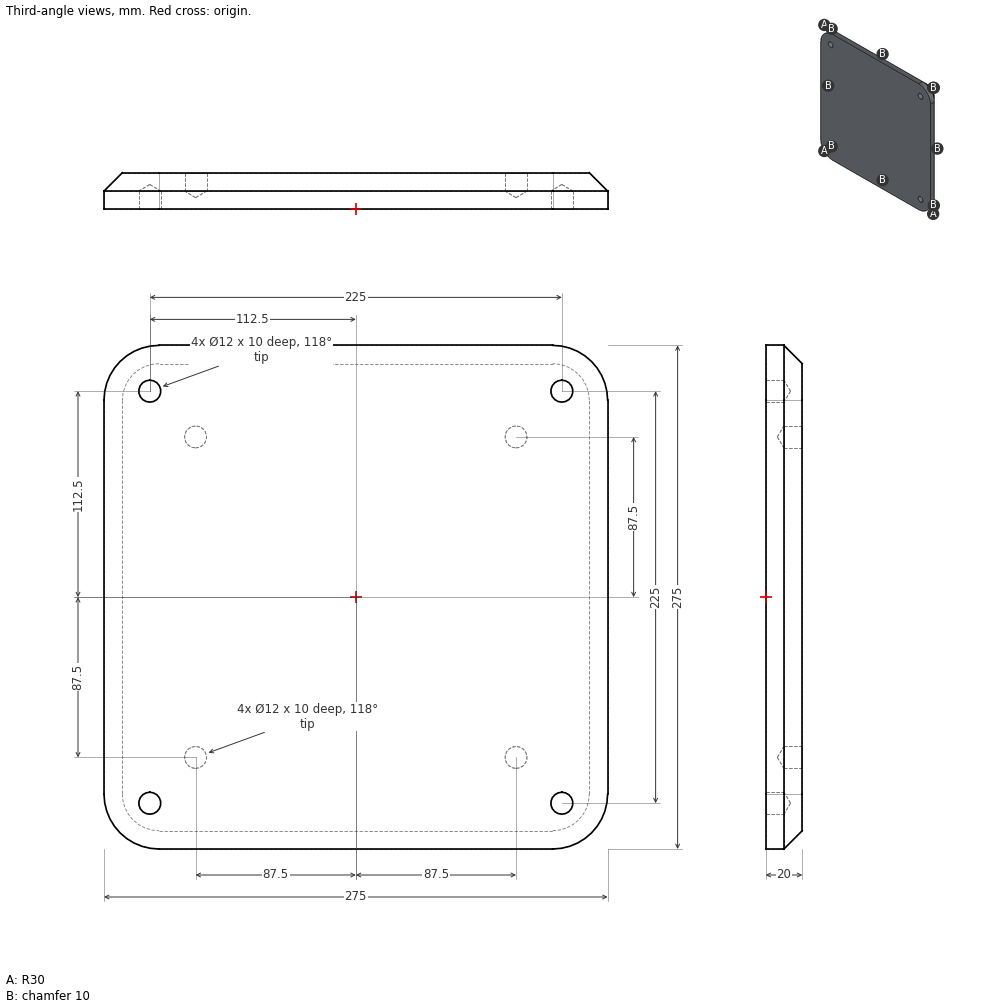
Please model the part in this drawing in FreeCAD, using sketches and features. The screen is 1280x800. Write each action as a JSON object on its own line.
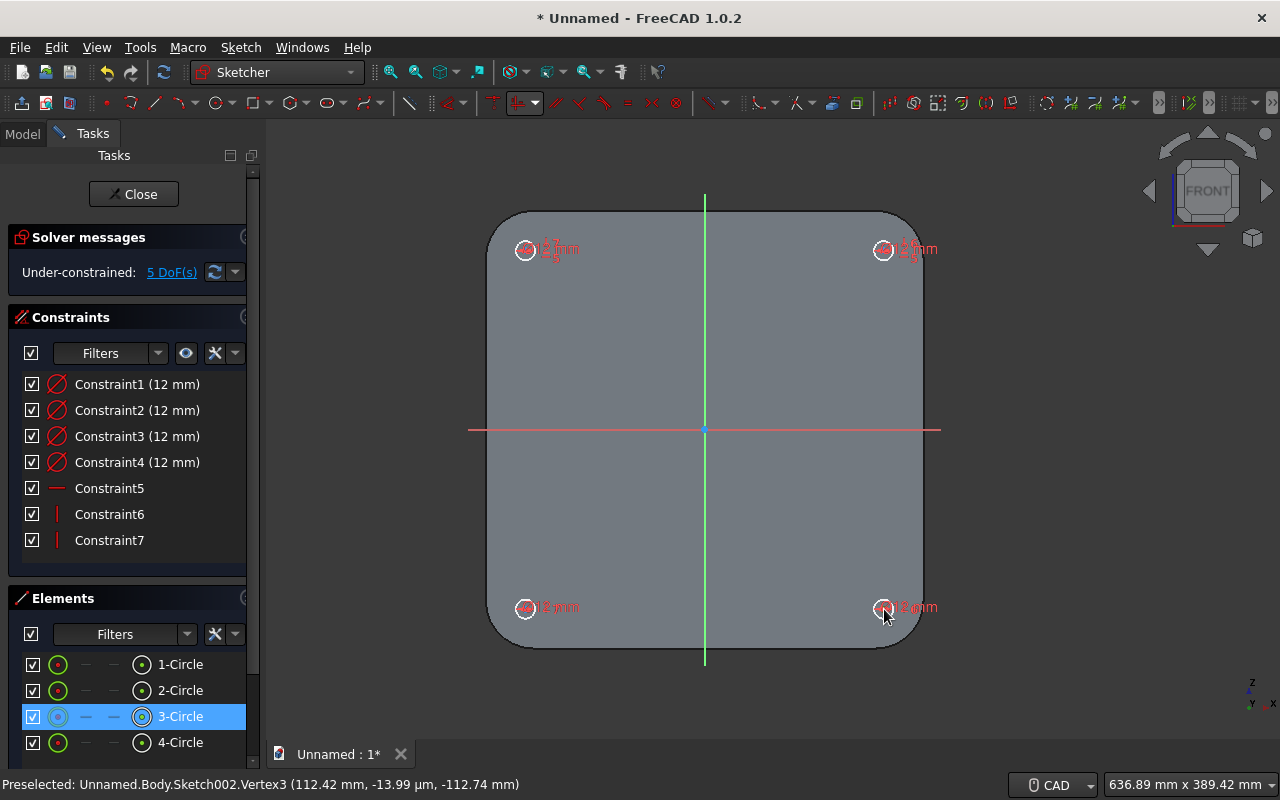
{"action": "left_click", "coordinate": [526, 609]}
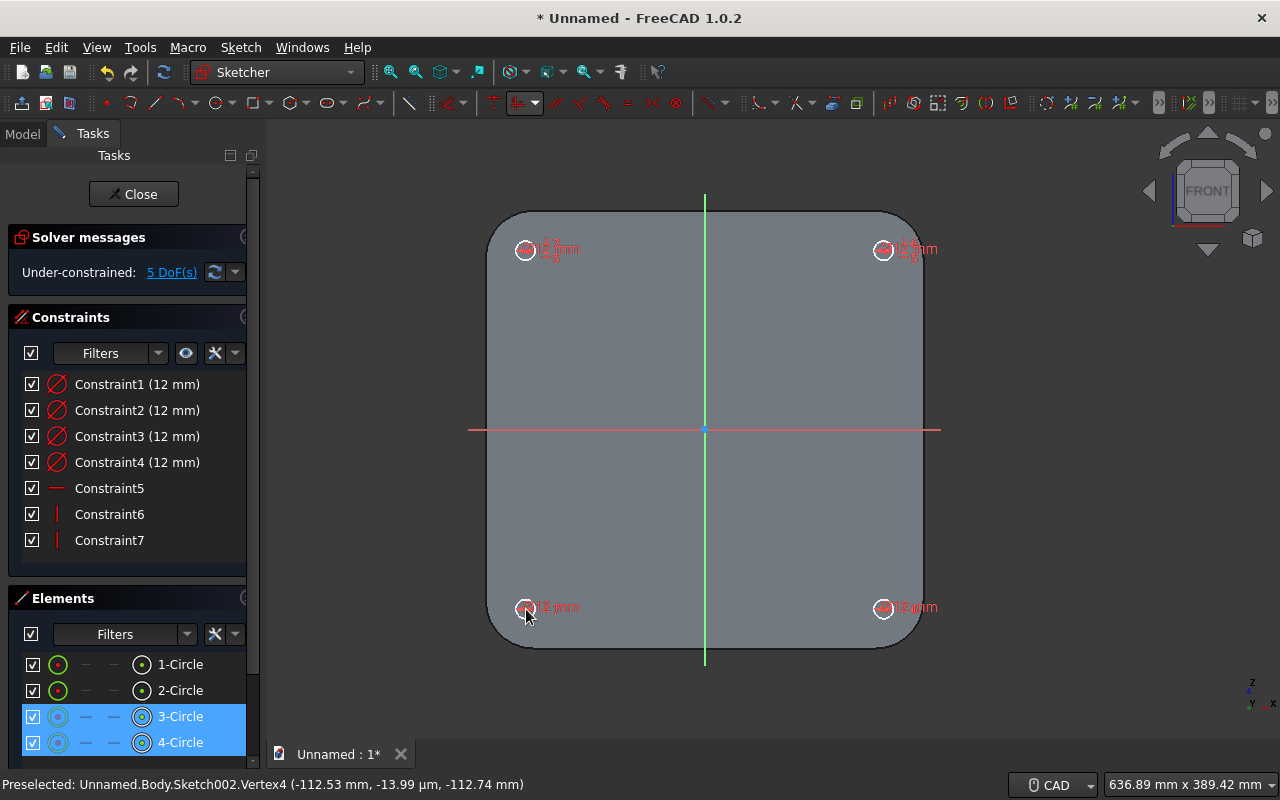
{"action": "key", "text": "h"}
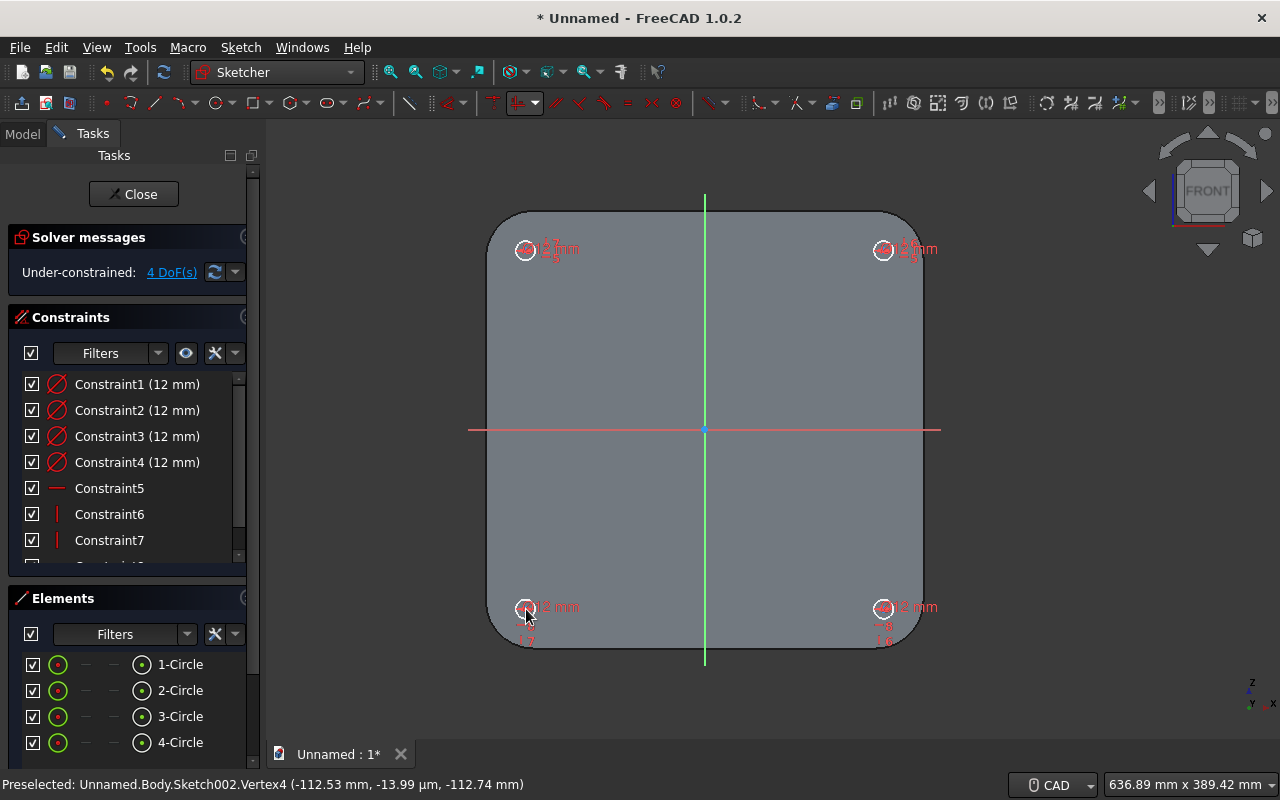
{"action": "key", "text": "d"}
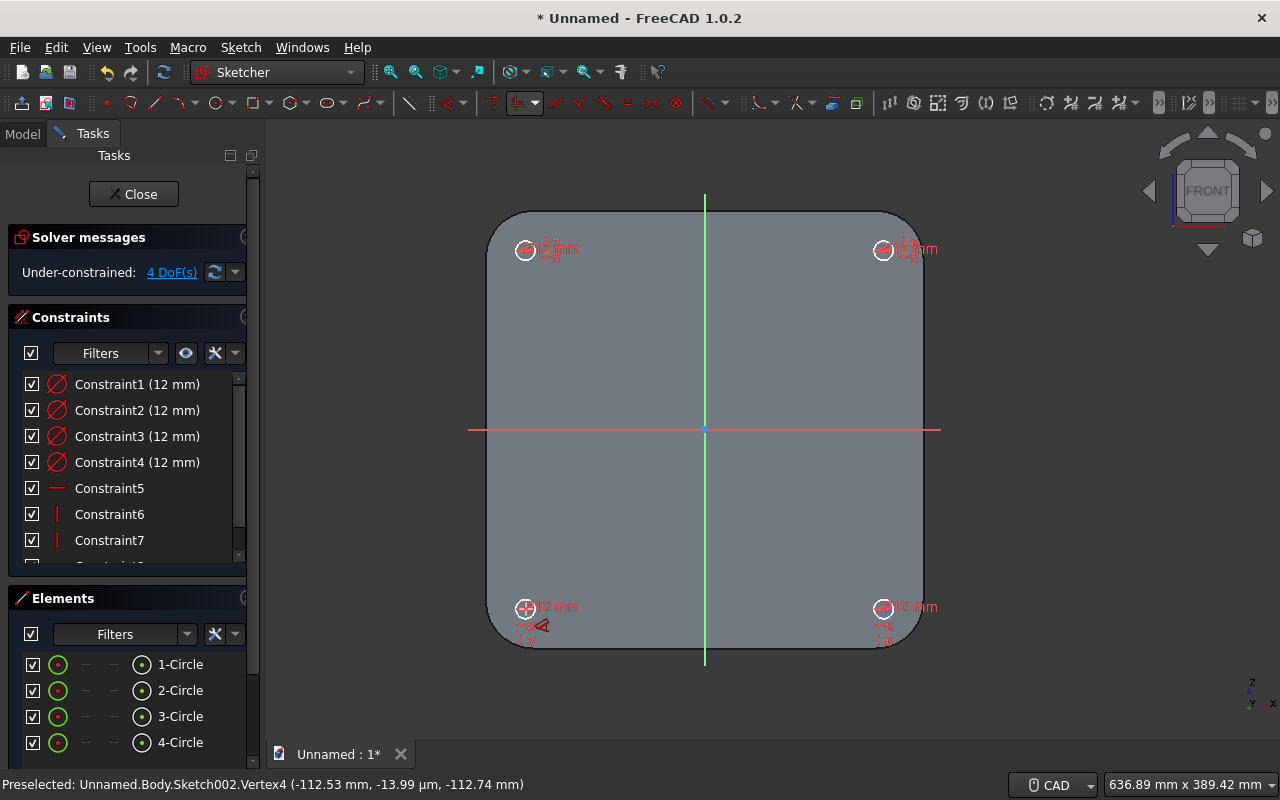
{"action": "left_click", "coordinate": [526, 251]}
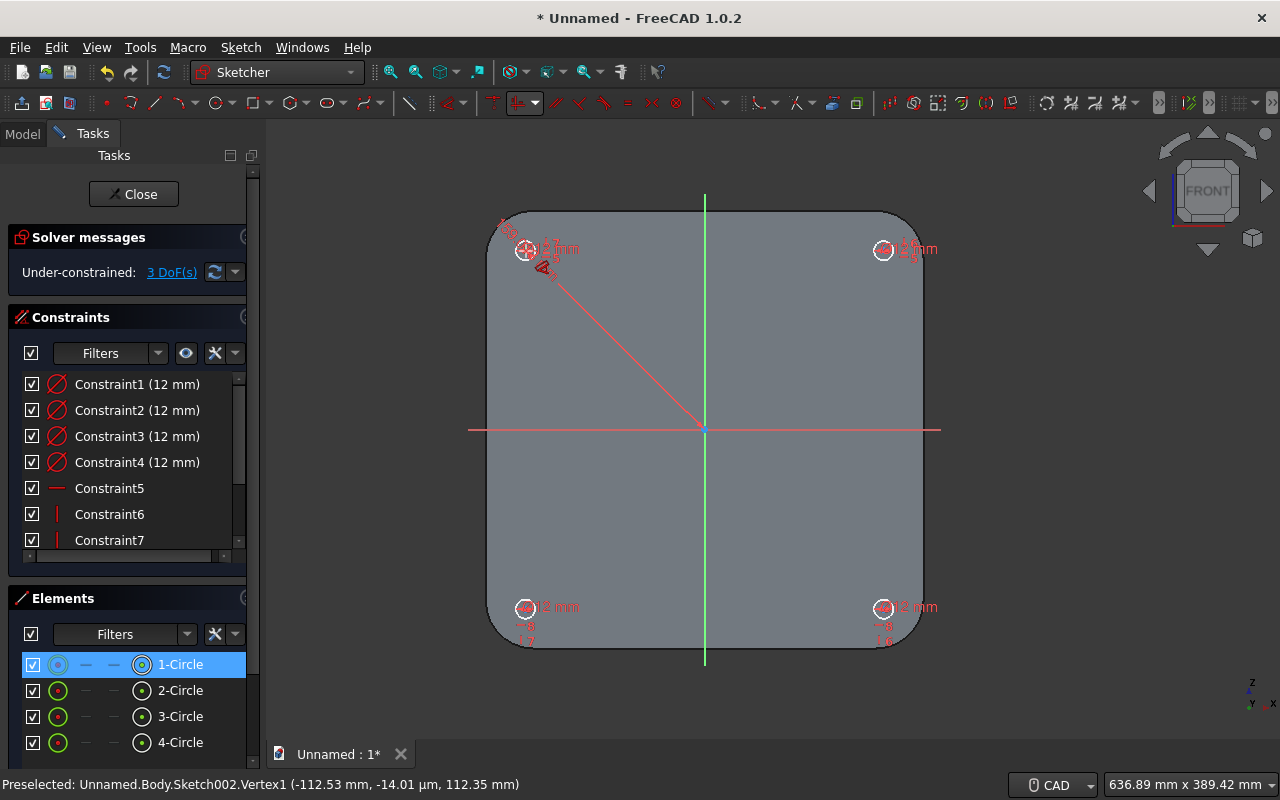
{"action": "left_click", "coordinate": [884, 251]}
{"action": "left_click", "coordinate": [622, 217]}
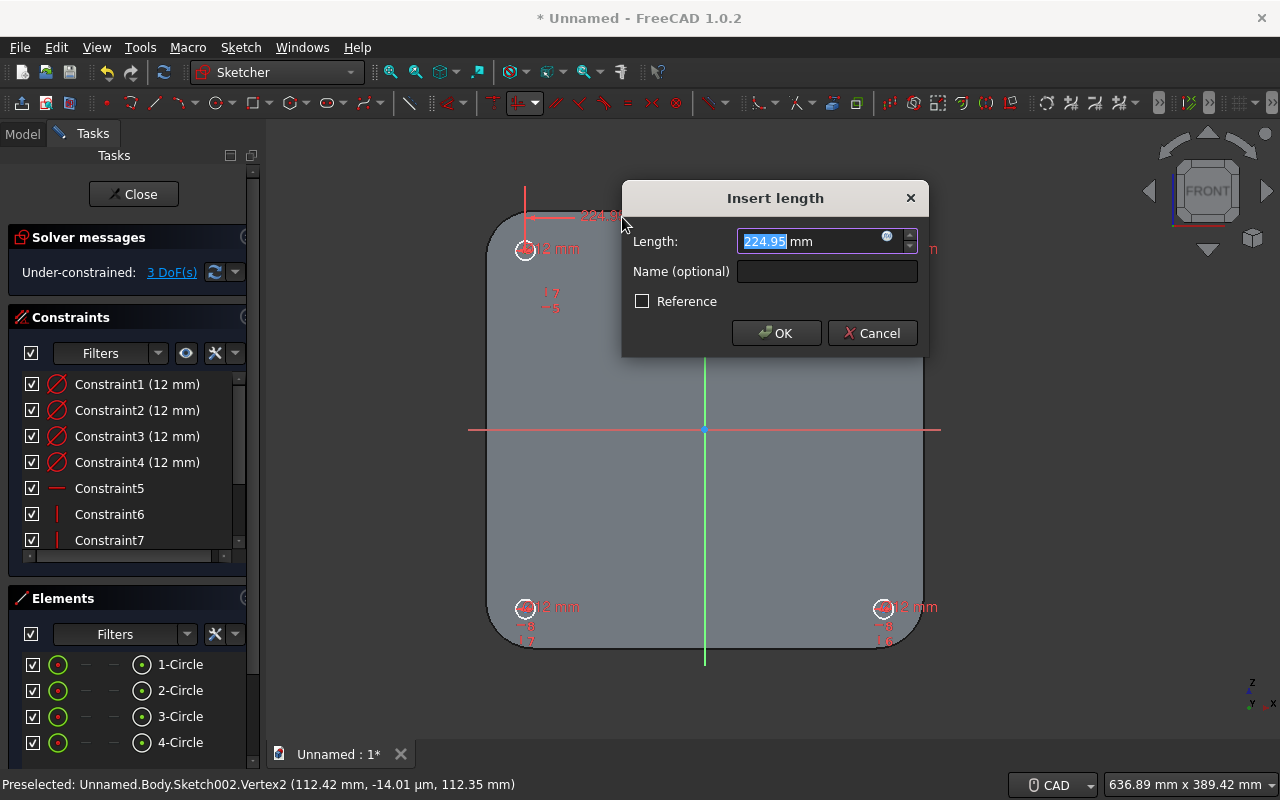
{"action": "type", "text": "225"}
{"action": "key", "text": "Return"}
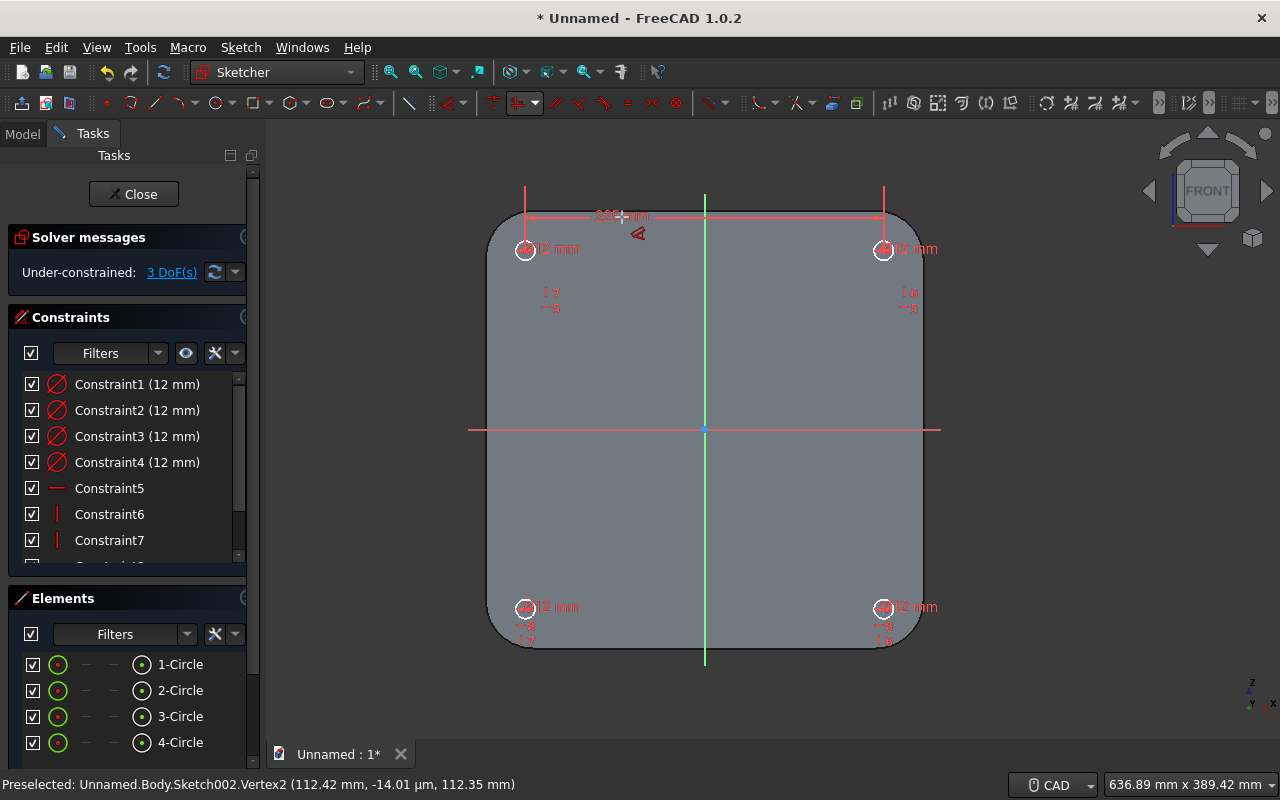
{"action": "left_click", "coordinate": [884, 251]}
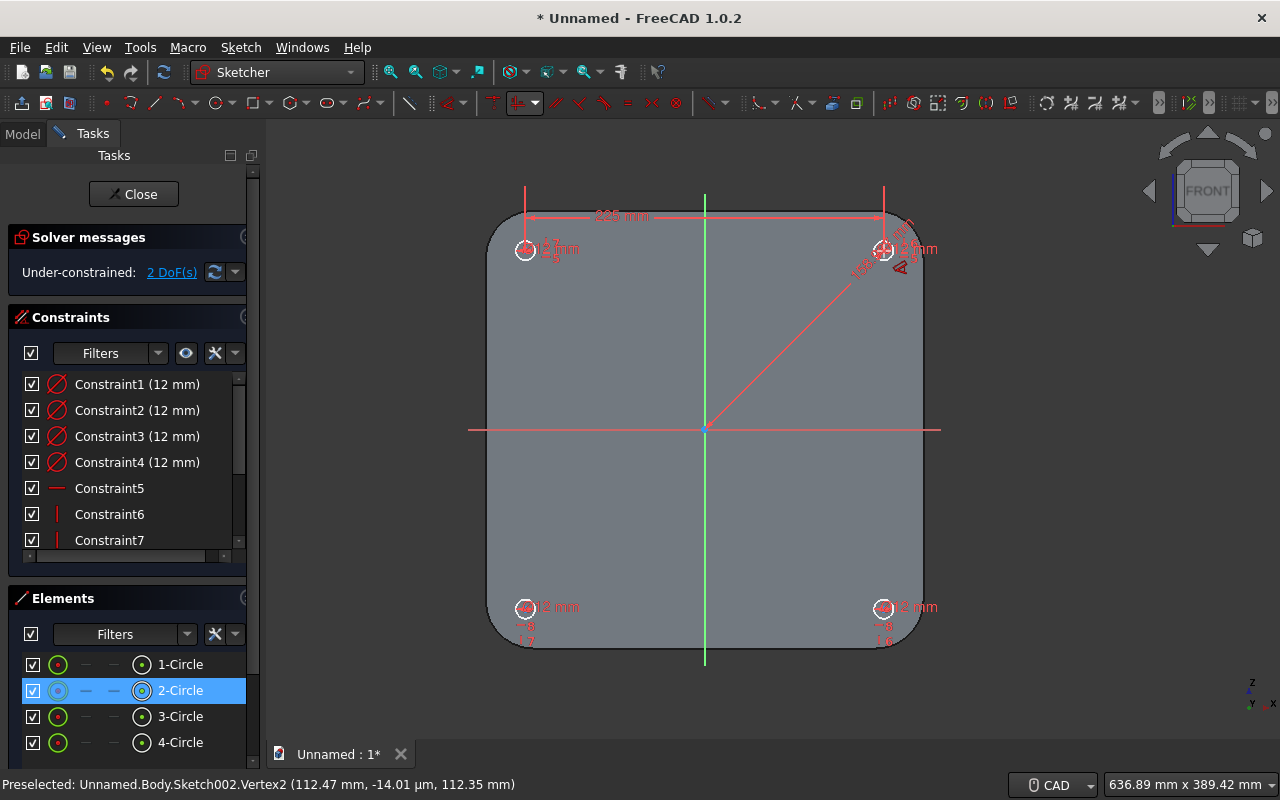
{"action": "left_click", "coordinate": [884, 609]}
{"action": "left_click", "coordinate": [918, 348]}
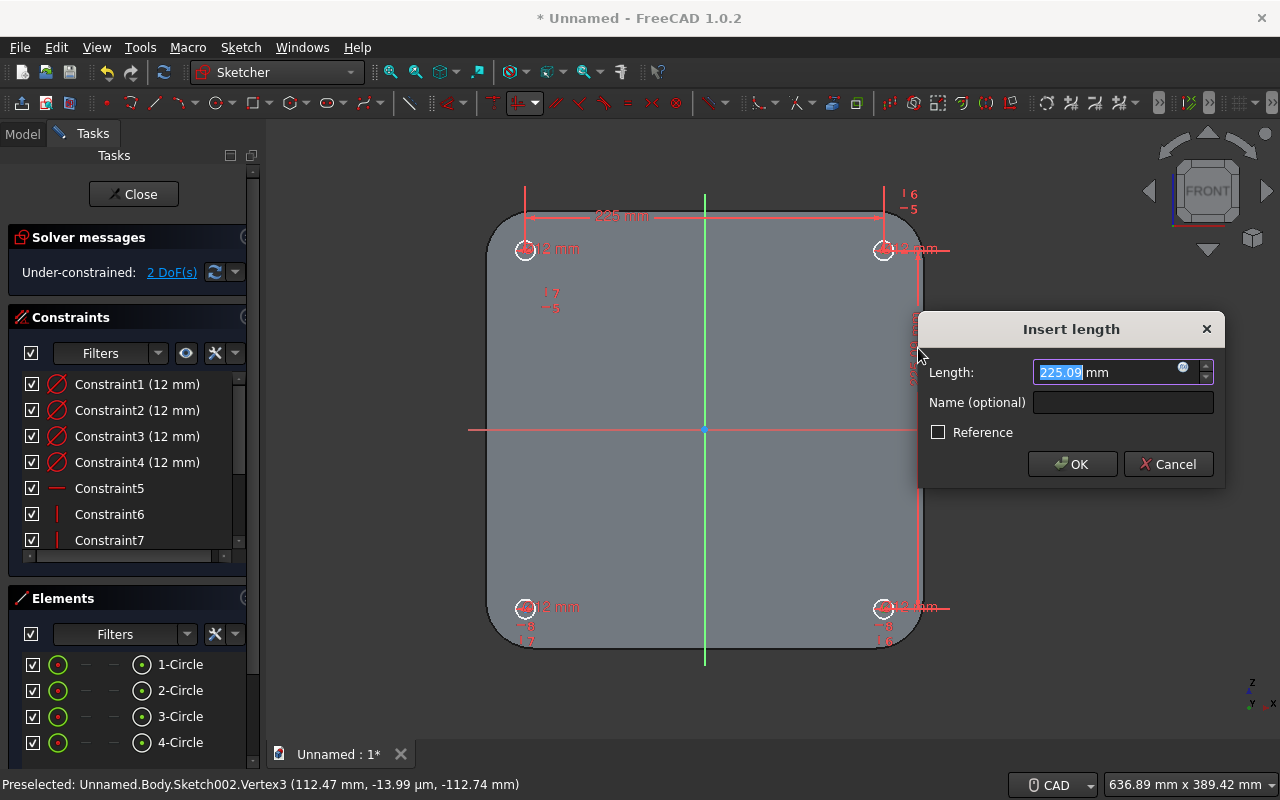
{"action": "type", "text": "225"}
{"action": "key", "text": "Return"}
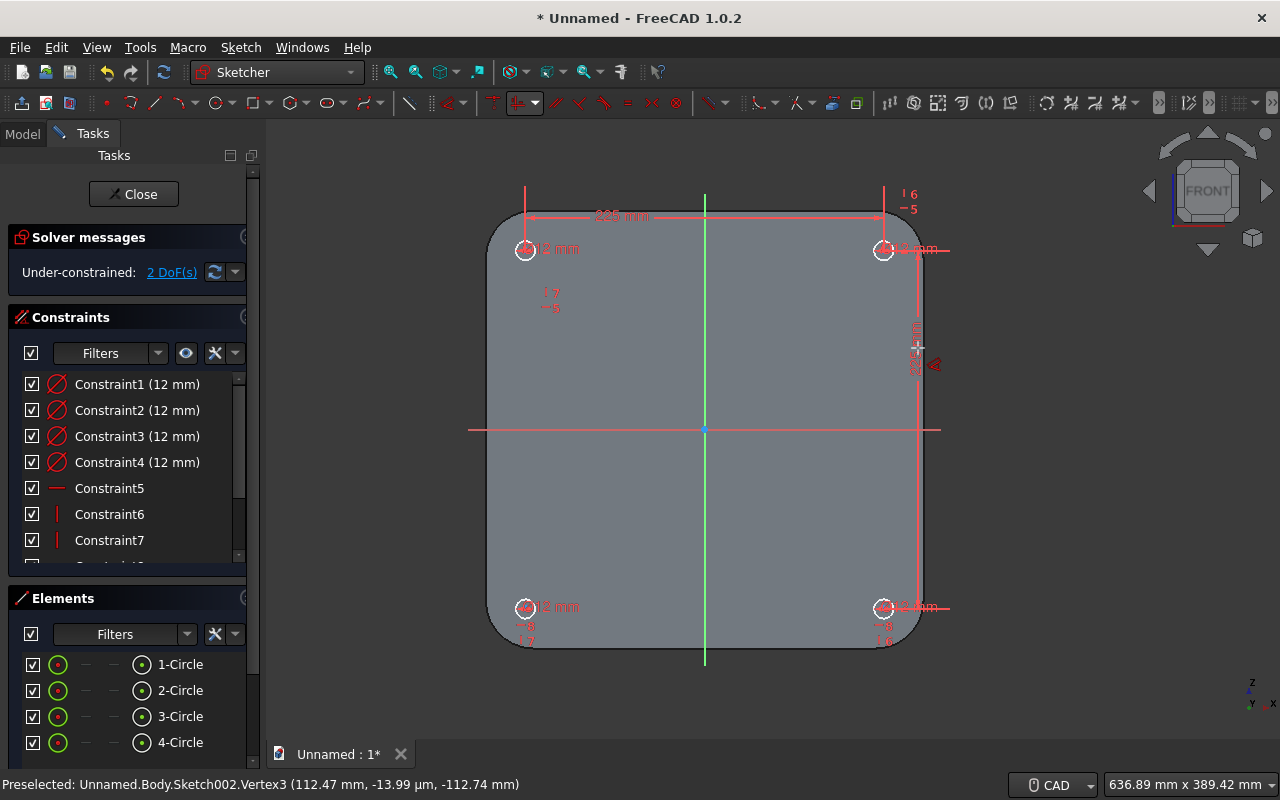
{"action": "left_click", "coordinate": [526, 251]}
{"action": "left_click", "coordinate": [615, 464]}